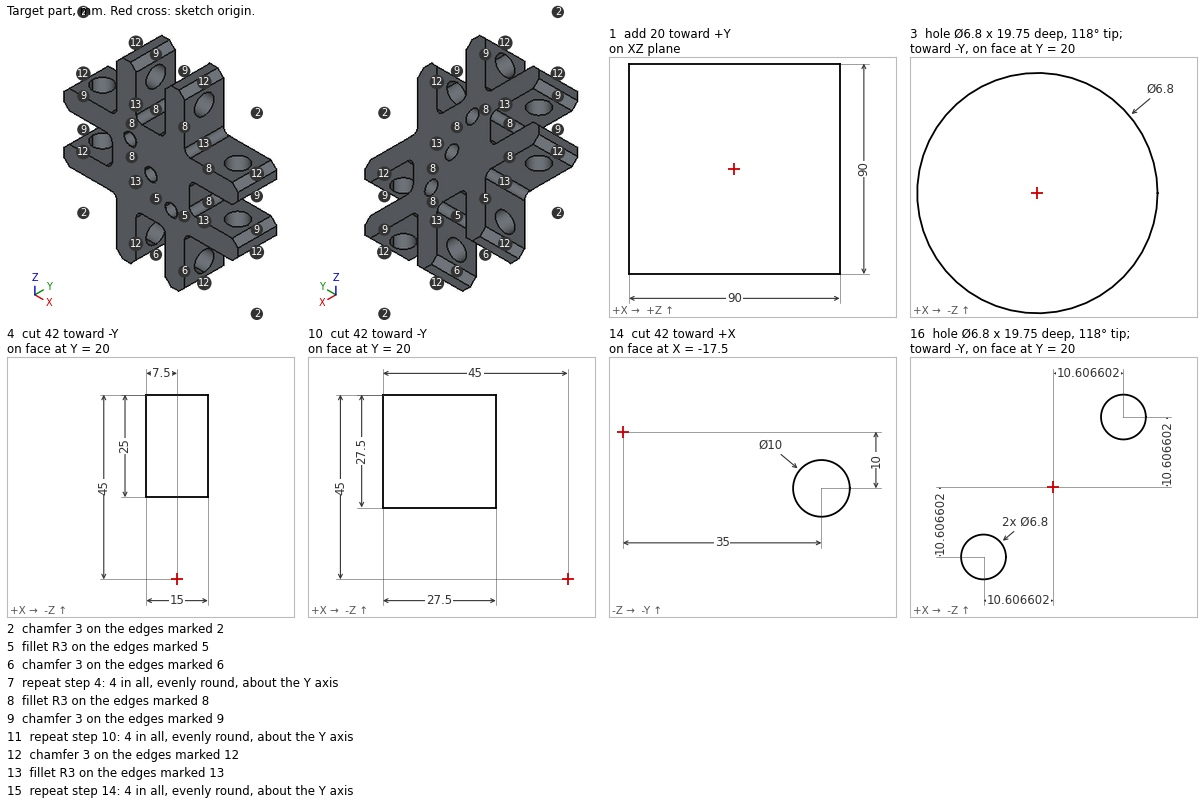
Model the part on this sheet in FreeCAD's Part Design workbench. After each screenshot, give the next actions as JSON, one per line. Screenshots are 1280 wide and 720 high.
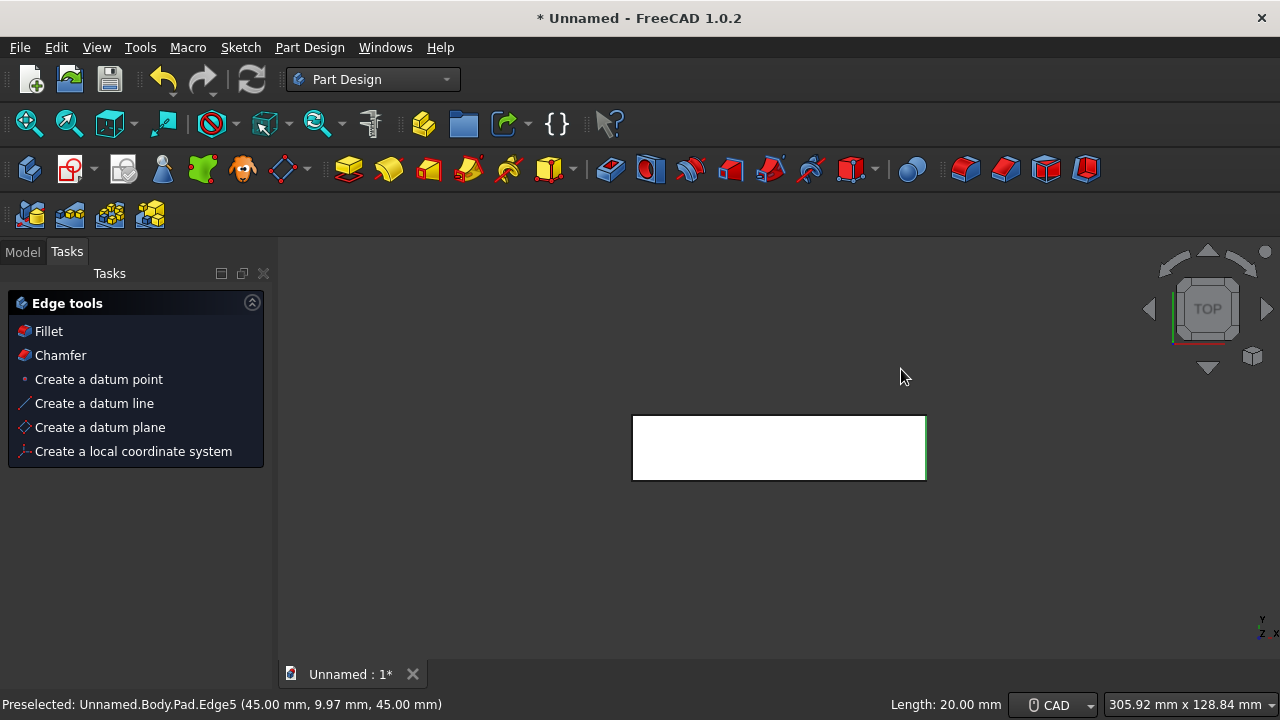
{"action": "left_click", "coordinate": [30, 124]}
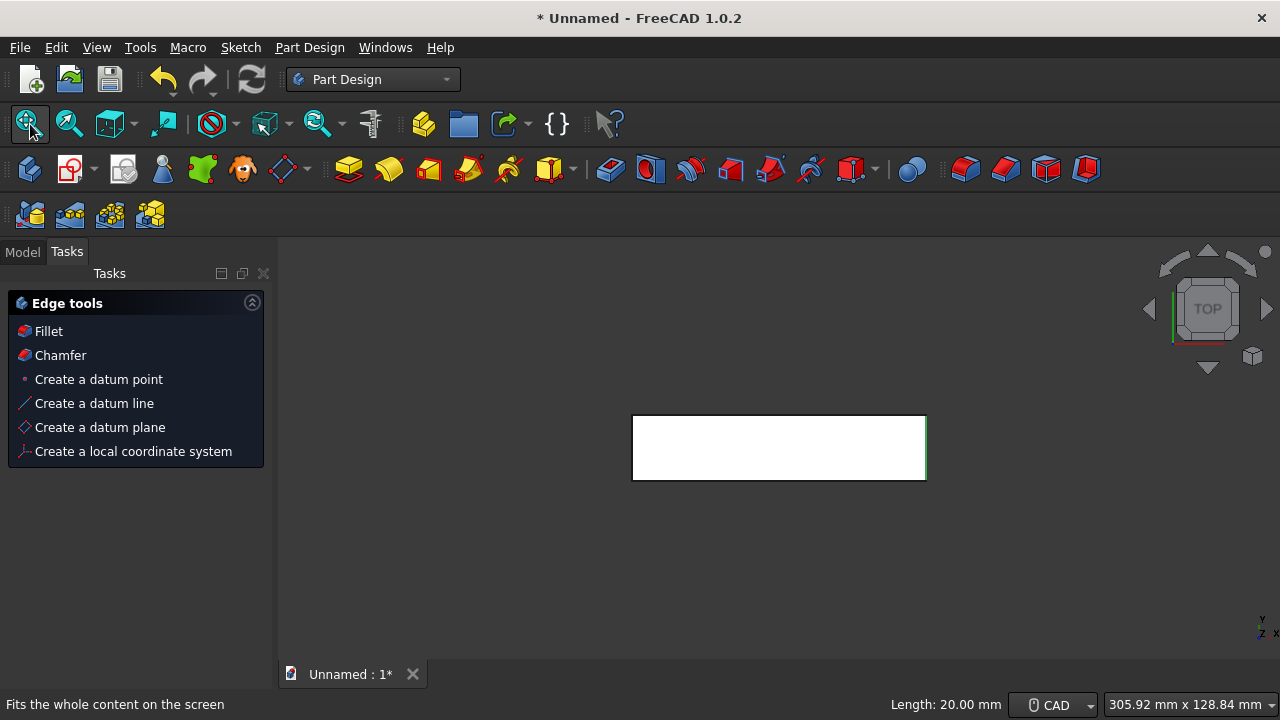
{"action": "left_click", "coordinate": [632, 447], "text": "ctrl"}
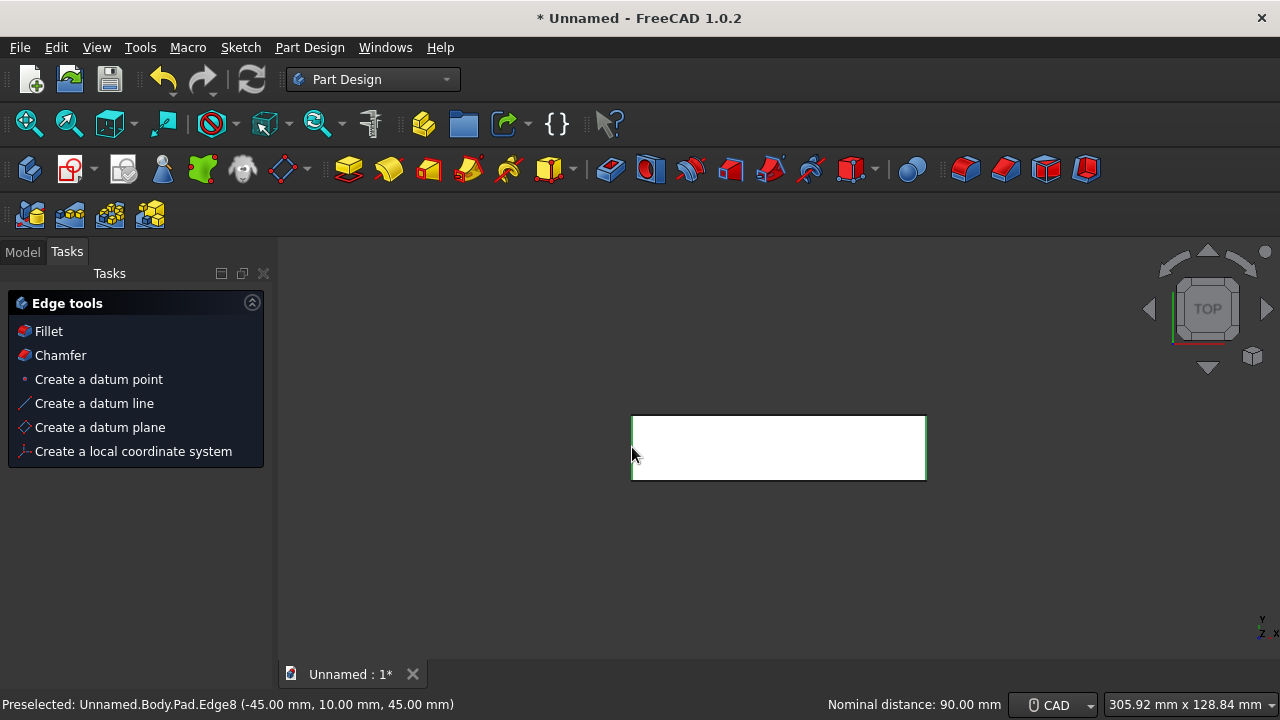
{"action": "key", "text": "1"}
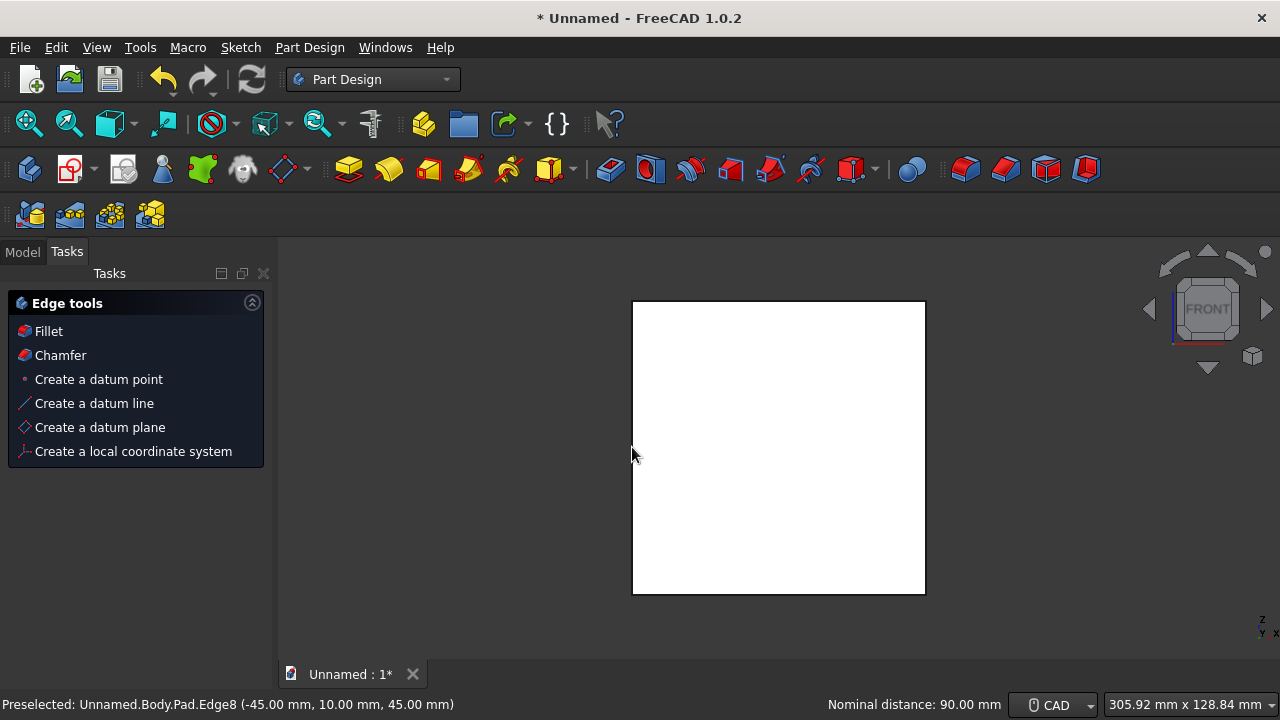
{"action": "key", "text": "3"}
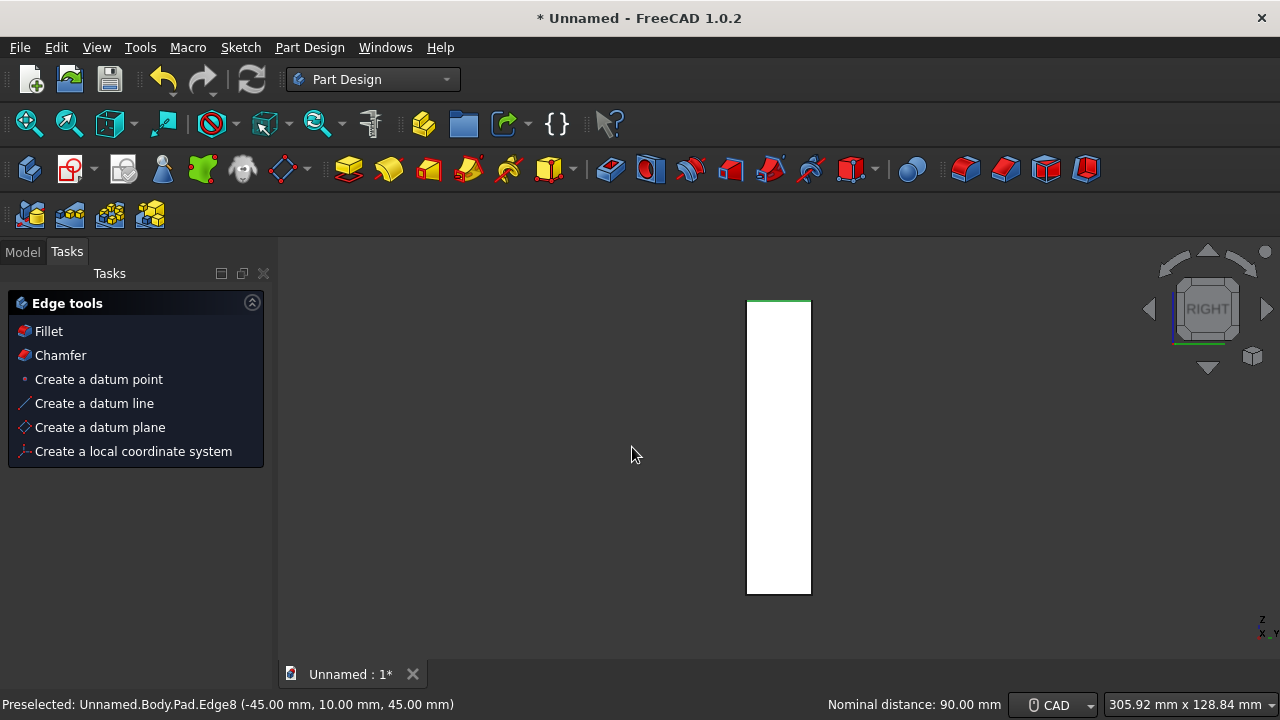
{"action": "left_click", "coordinate": [779, 594], "text": "ctrl"}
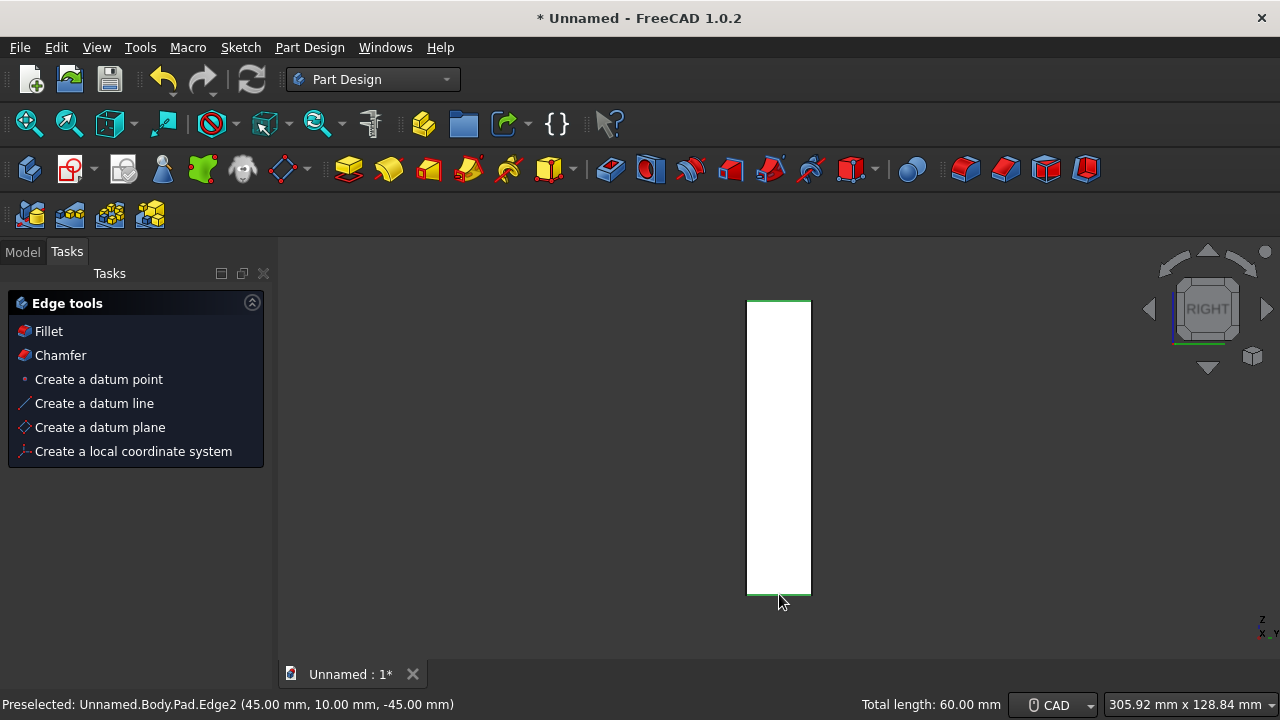
{"action": "key", "text": "5"}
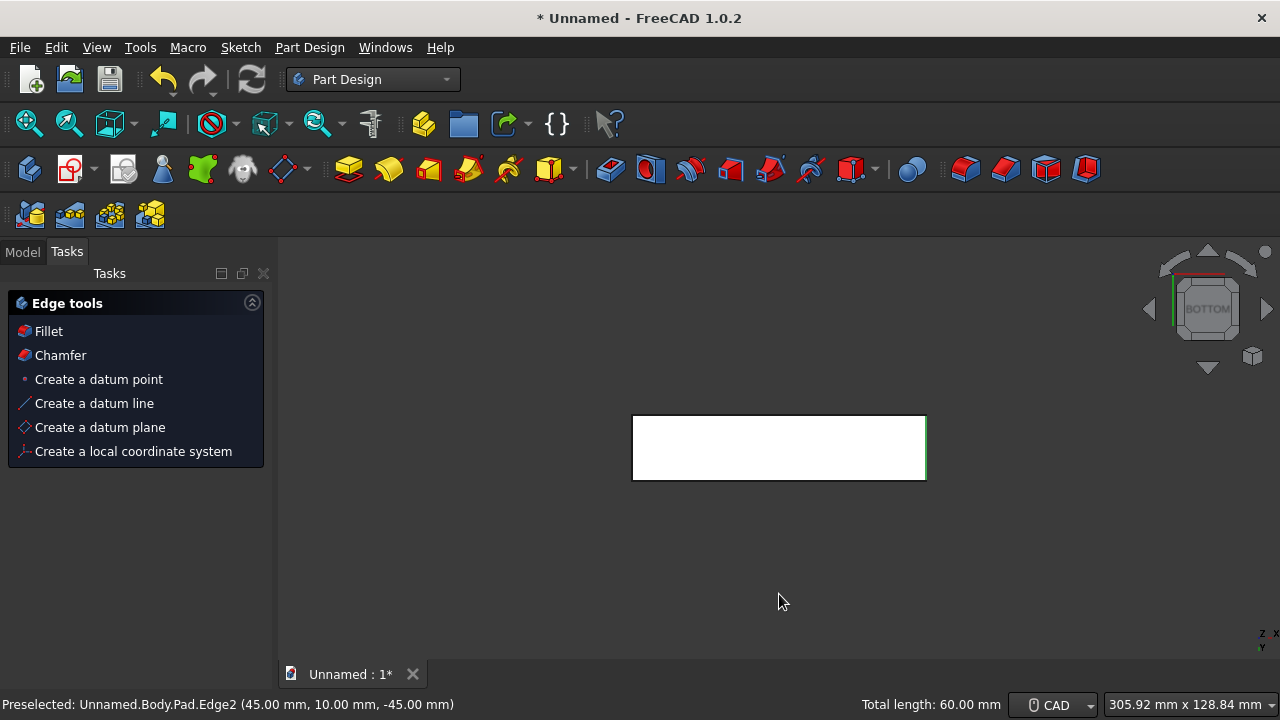
{"action": "left_click", "coordinate": [30, 124]}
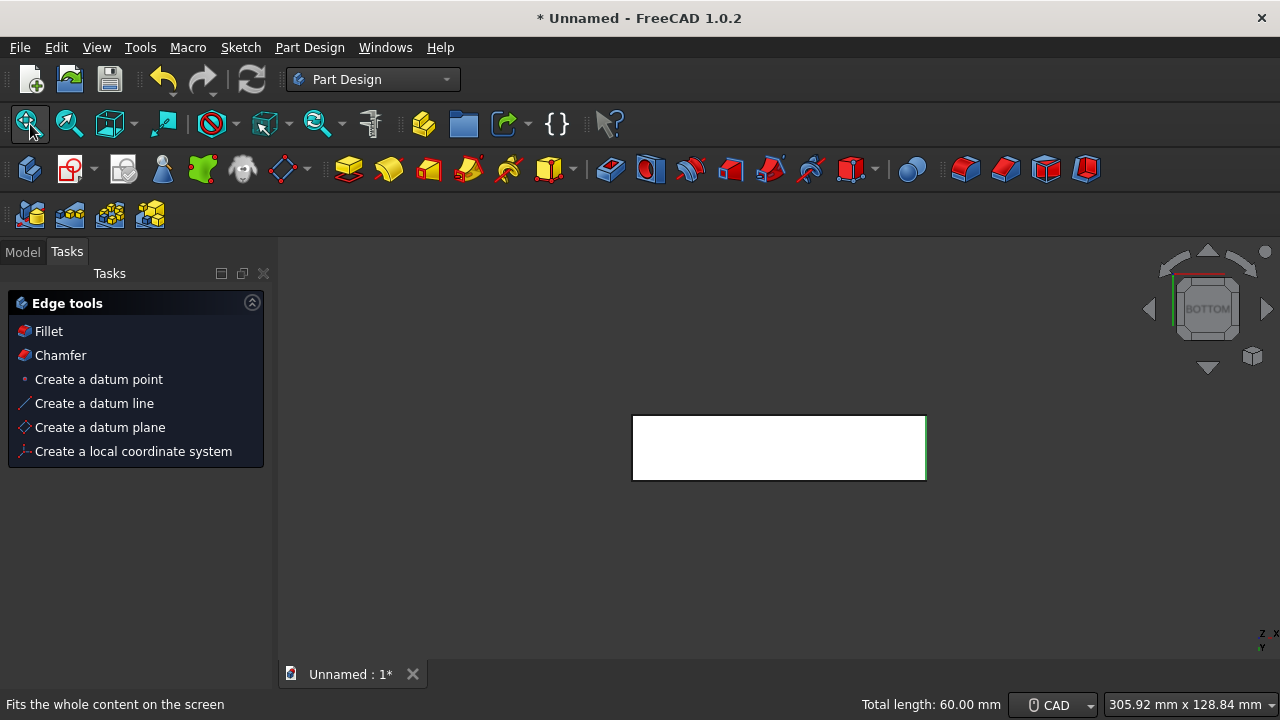
{"action": "left_click", "coordinate": [632, 447], "text": "ctrl"}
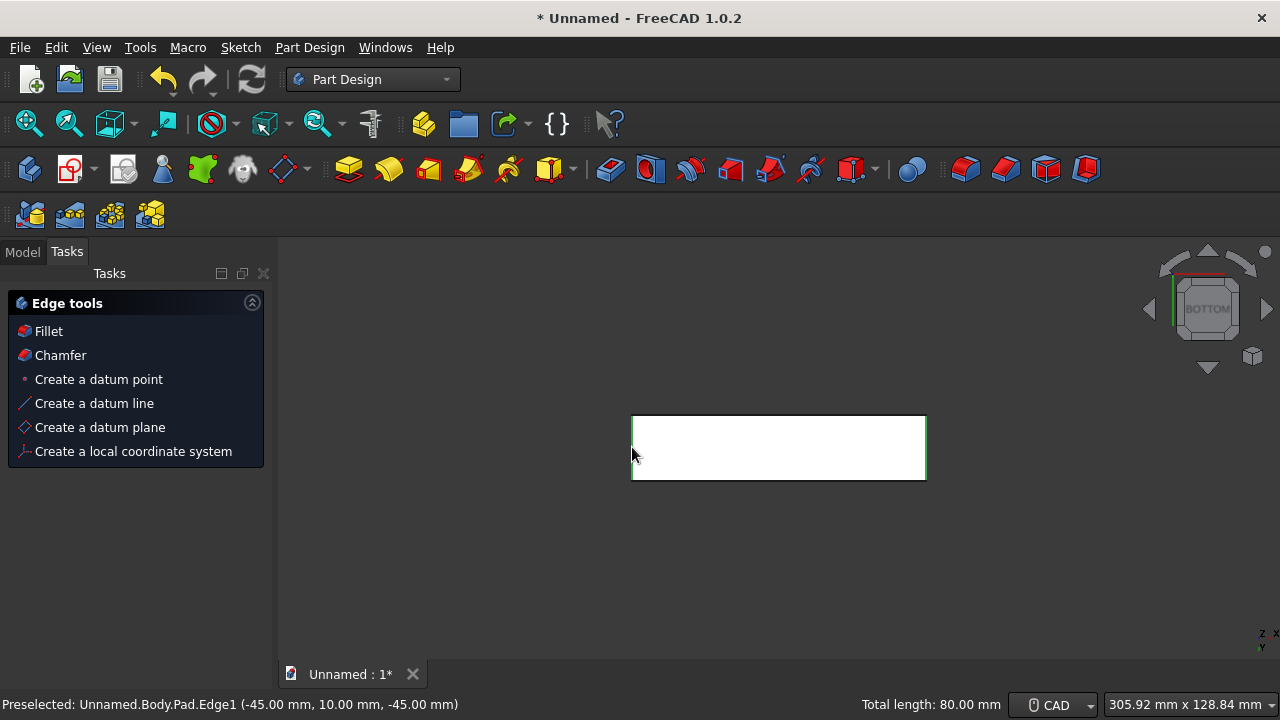
{"action": "left_click", "coordinate": [1006, 170]}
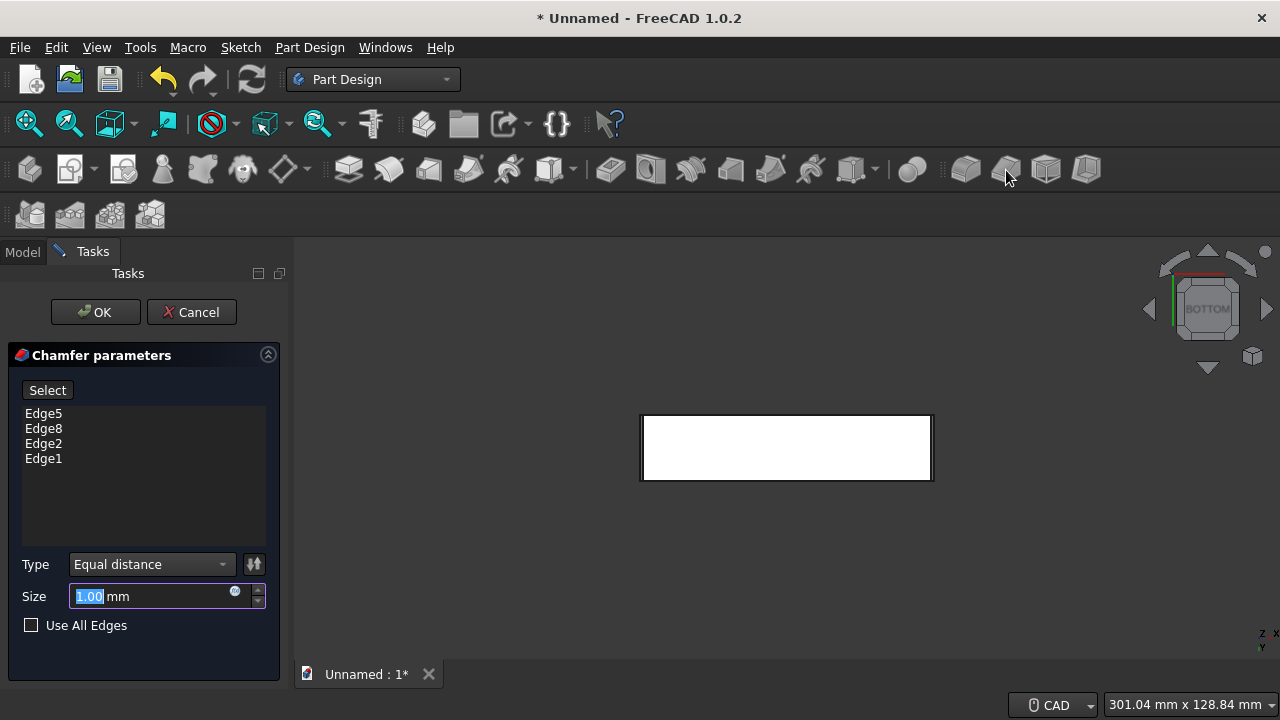
{"action": "type", "text": "3"}
{"action": "key", "text": "Tab"}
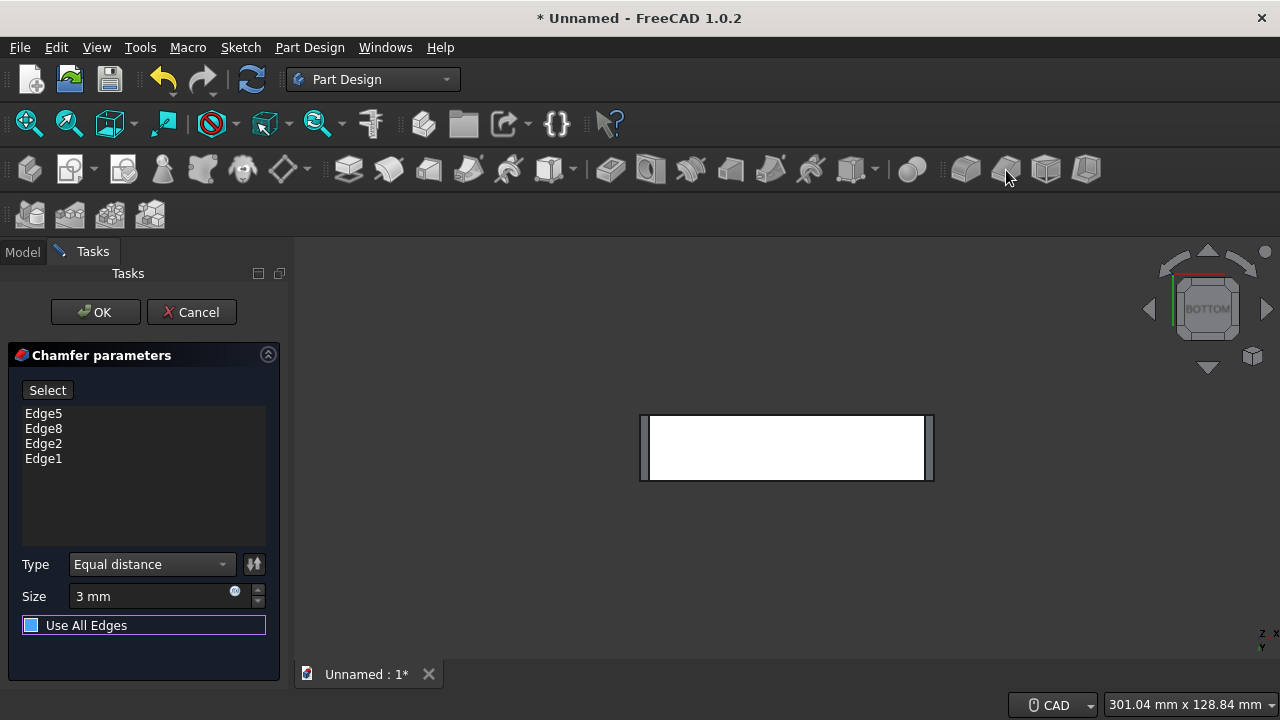
{"action": "left_click", "coordinate": [96, 312]}